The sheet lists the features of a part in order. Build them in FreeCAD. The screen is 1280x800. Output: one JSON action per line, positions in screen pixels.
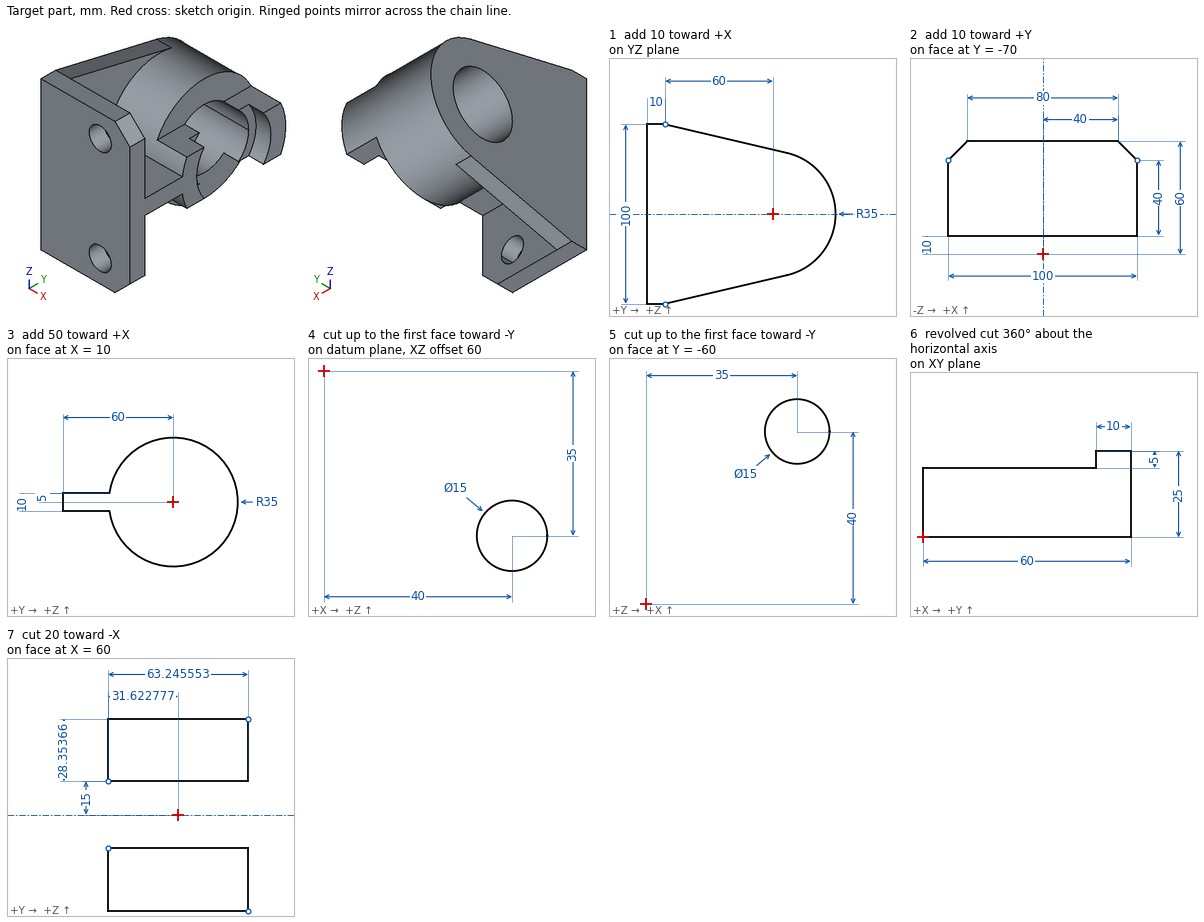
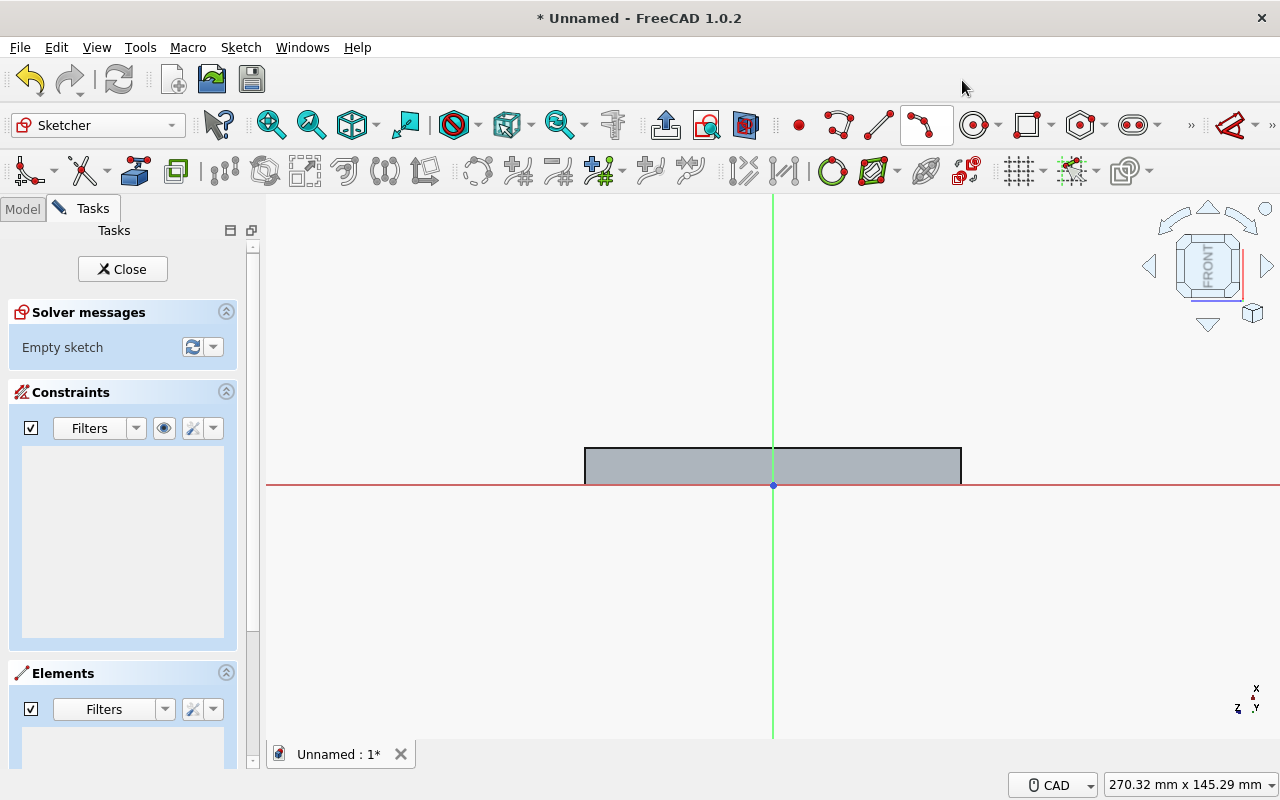
{"action": "scroll", "coordinate": [912, 222], "scroll_direction": "up", "scroll_amount": 2}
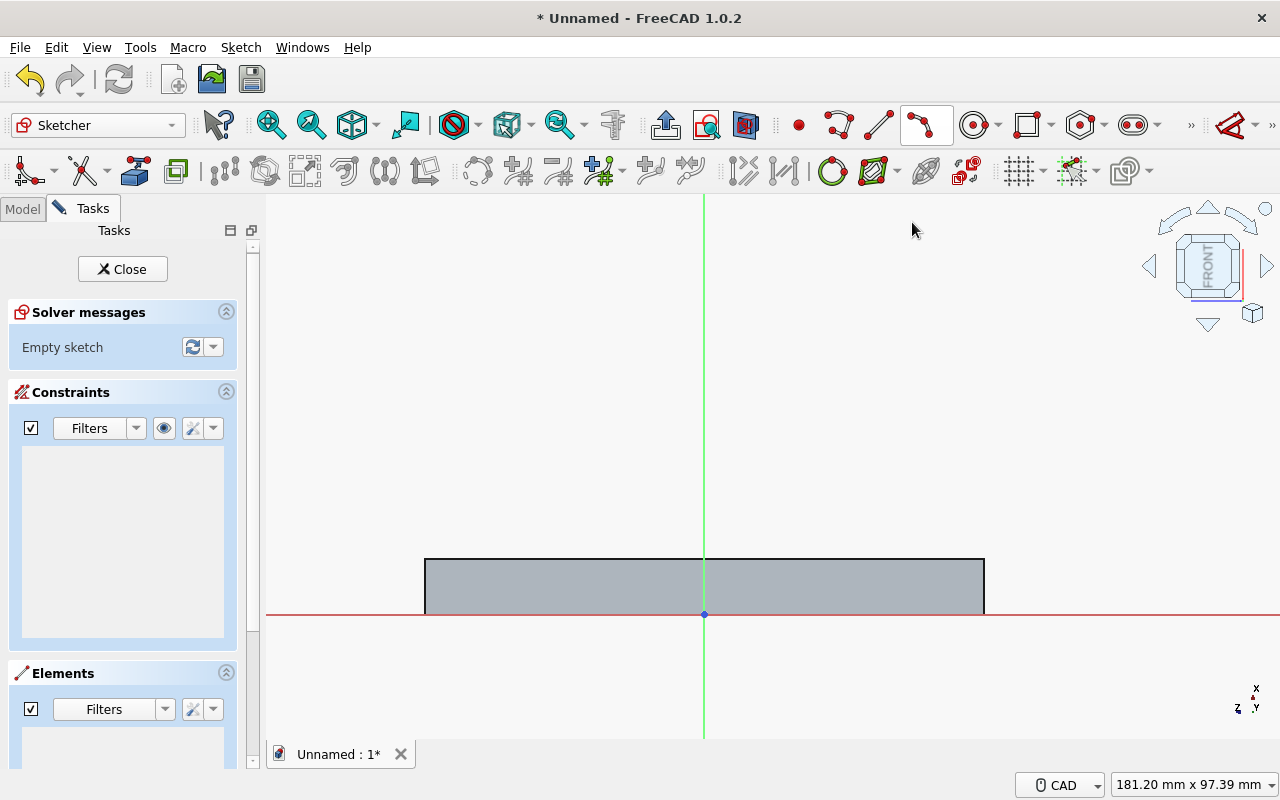
{"action": "key", "text": "g m"}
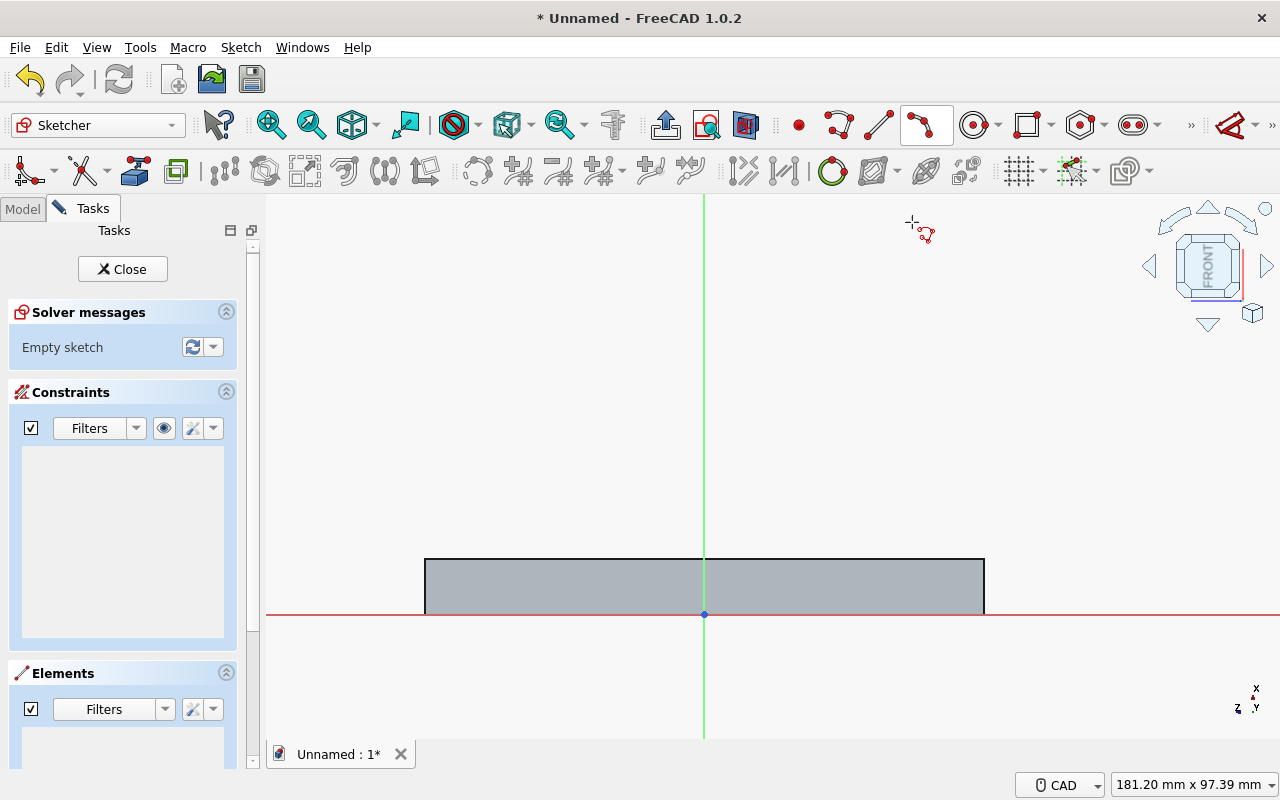
{"action": "left_click", "coordinate": [425, 559]}
{"action": "left_click", "coordinate": [984, 559]}
{"action": "left_click", "coordinate": [984, 335]}
{"action": "left_click", "coordinate": [928, 279]}
{"action": "left_click", "coordinate": [480, 279]}
{"action": "left_click", "coordinate": [425, 335]}
{"action": "left_click", "coordinate": [425, 560]}
{"action": "key", "text": "Escape"}
{"action": "key", "text": "Escape"}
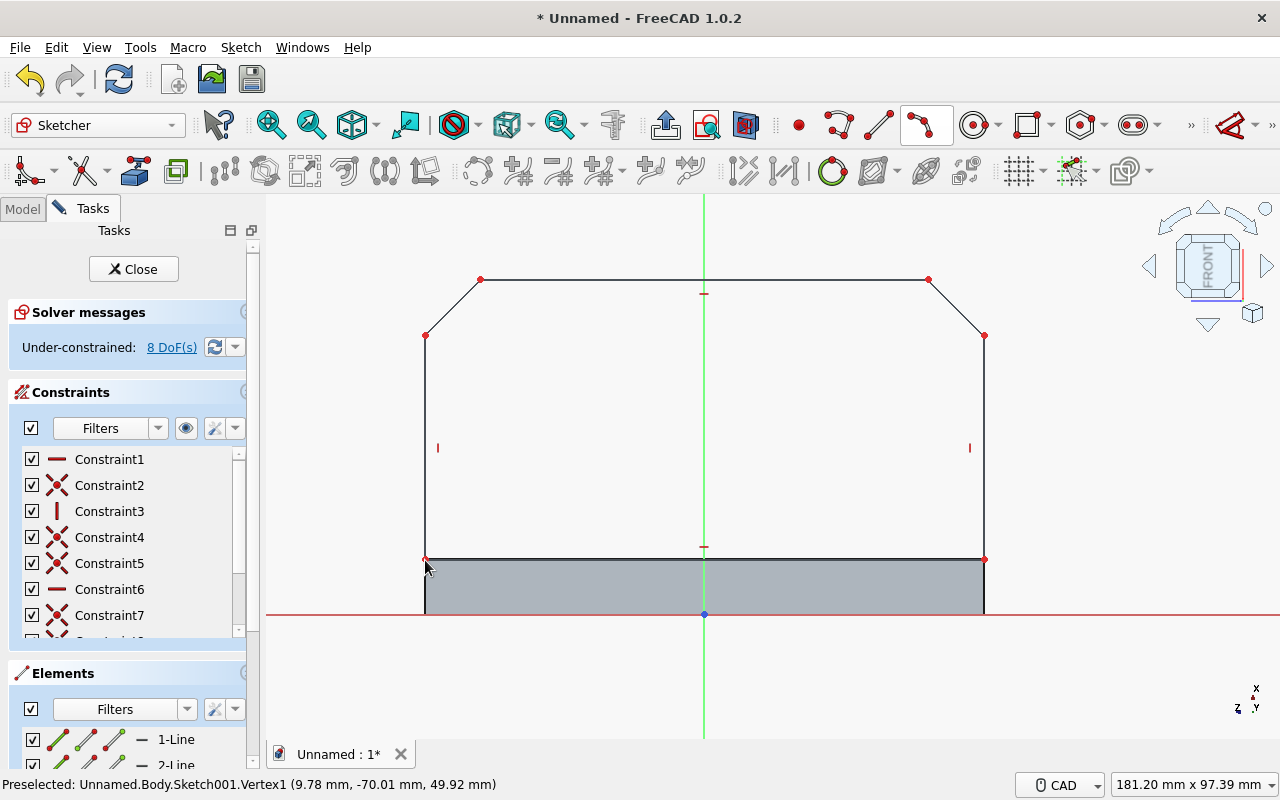
{"action": "left_click", "coordinate": [984, 336]}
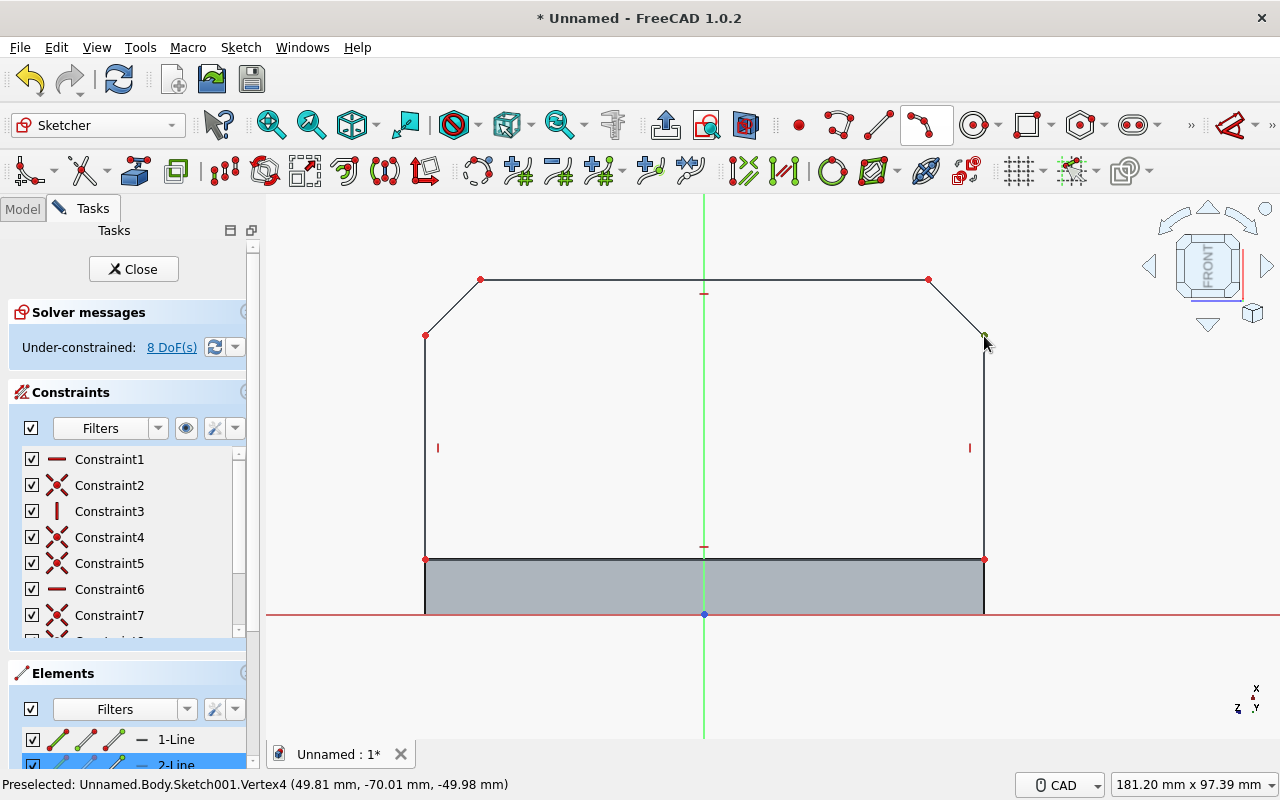
{"action": "left_click", "coordinate": [425, 336]}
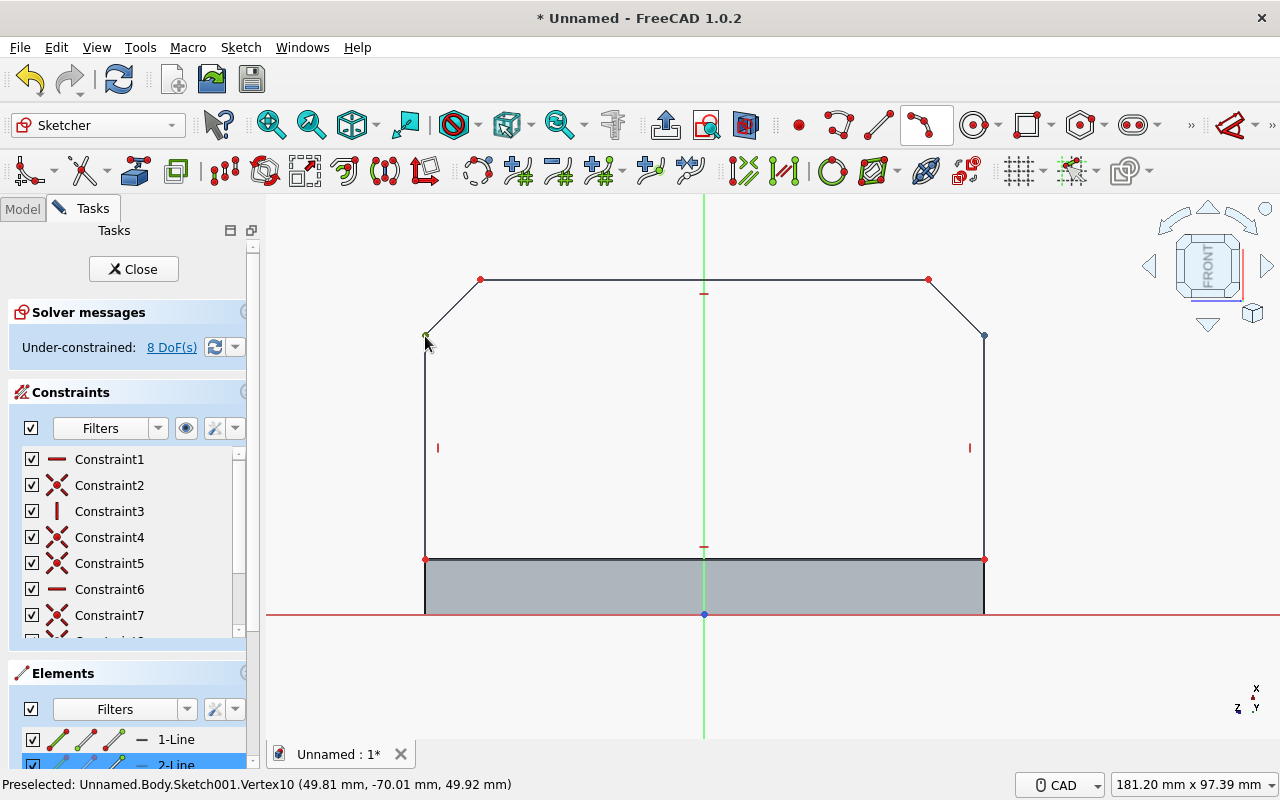
{"action": "left_click", "coordinate": [704, 676]}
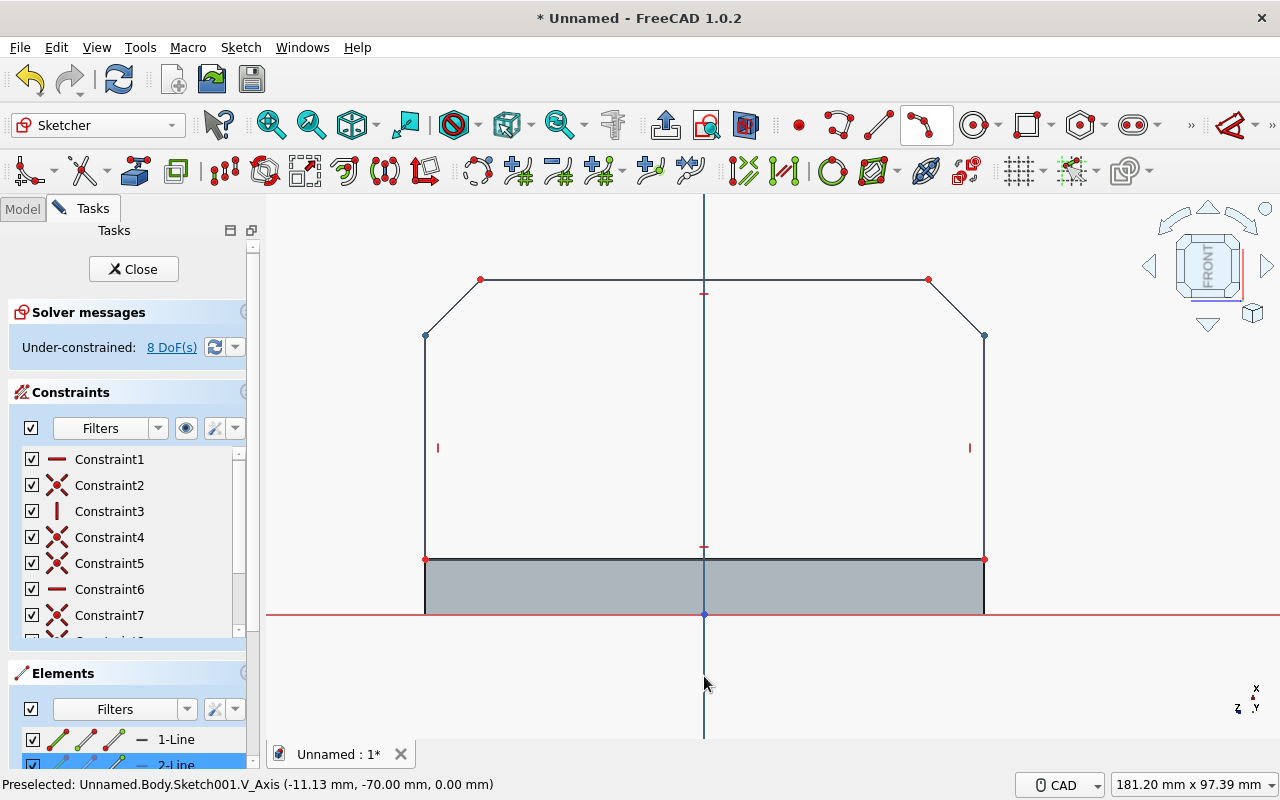
{"action": "key", "text": "s"}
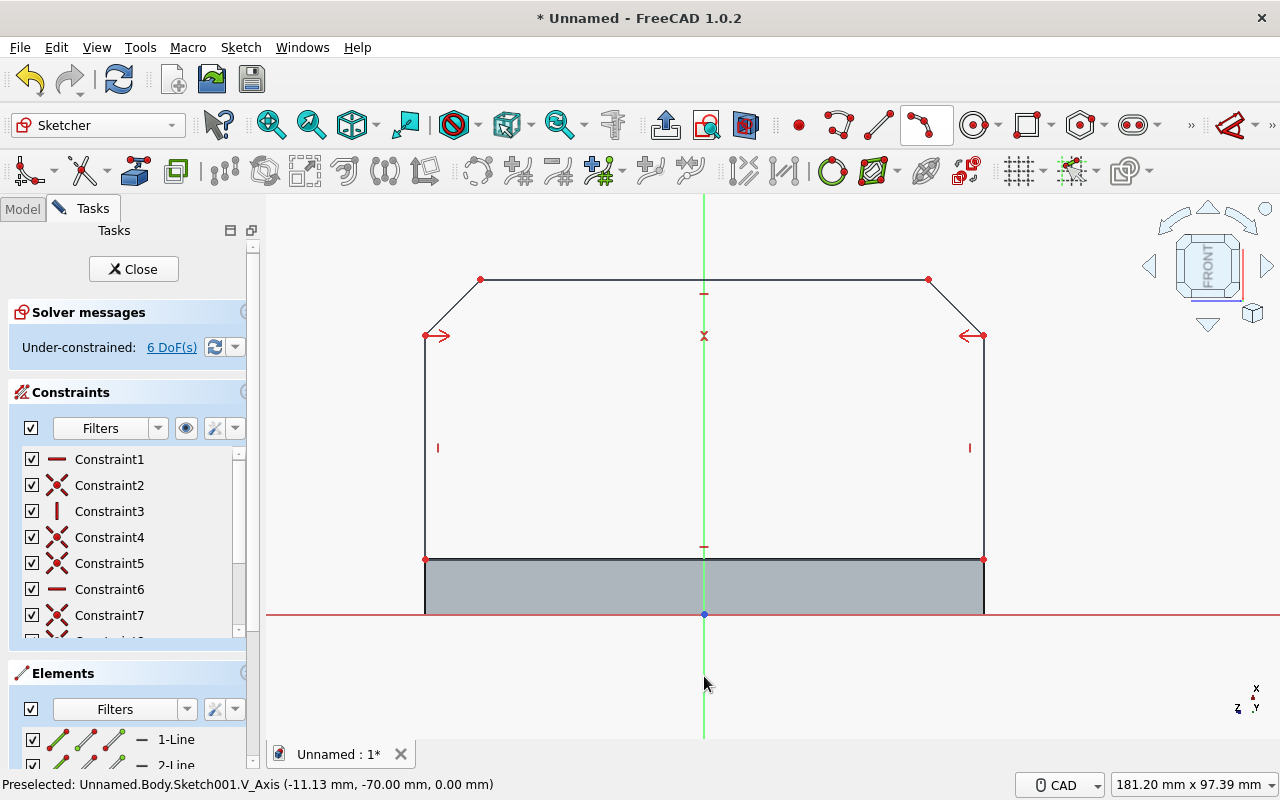
{"action": "left_click", "coordinate": [1230, 126]}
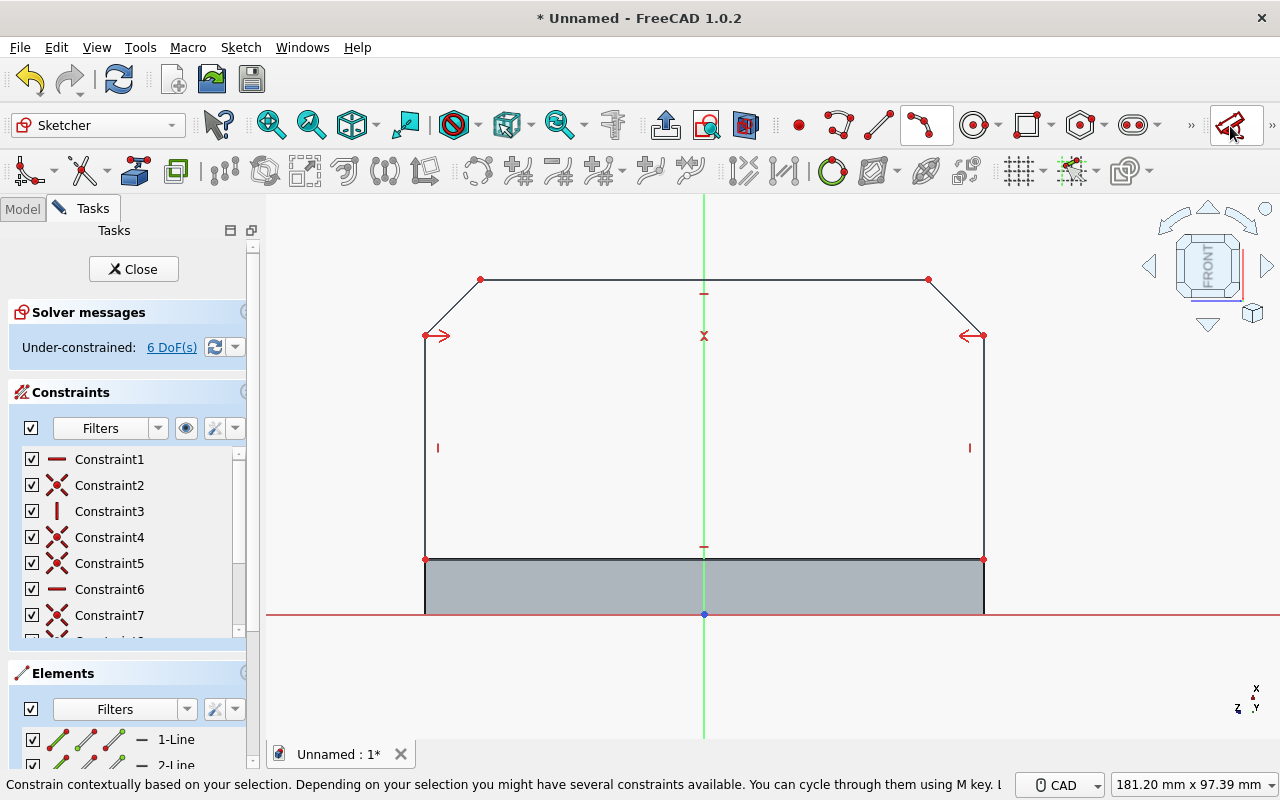
{"action": "left_click", "coordinate": [984, 493]}
{"action": "left_click", "coordinate": [1018, 448]}